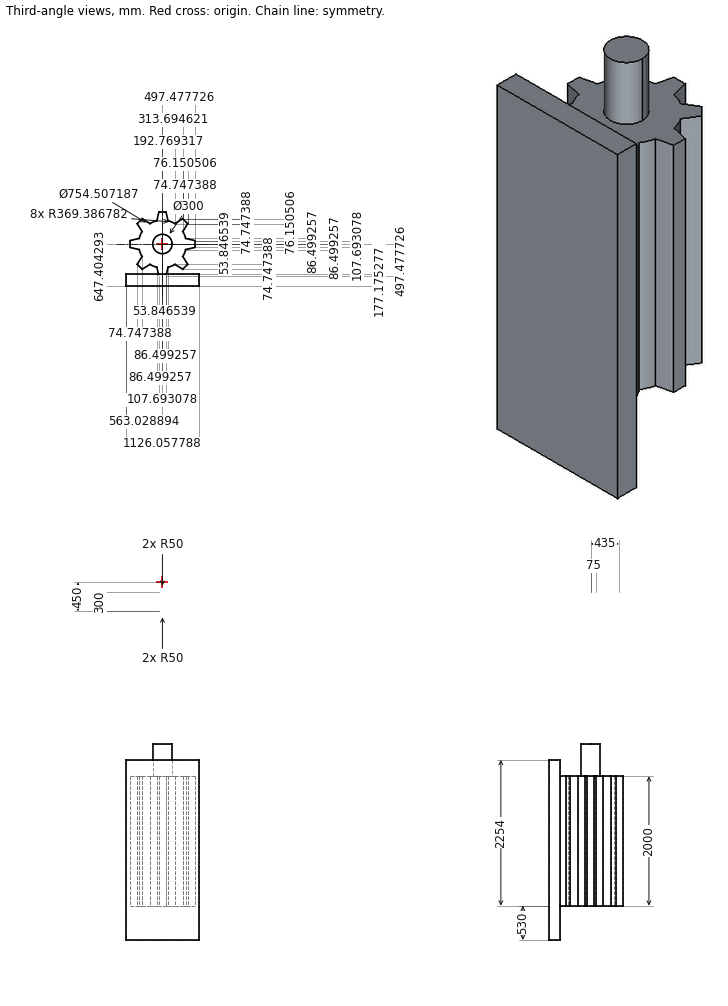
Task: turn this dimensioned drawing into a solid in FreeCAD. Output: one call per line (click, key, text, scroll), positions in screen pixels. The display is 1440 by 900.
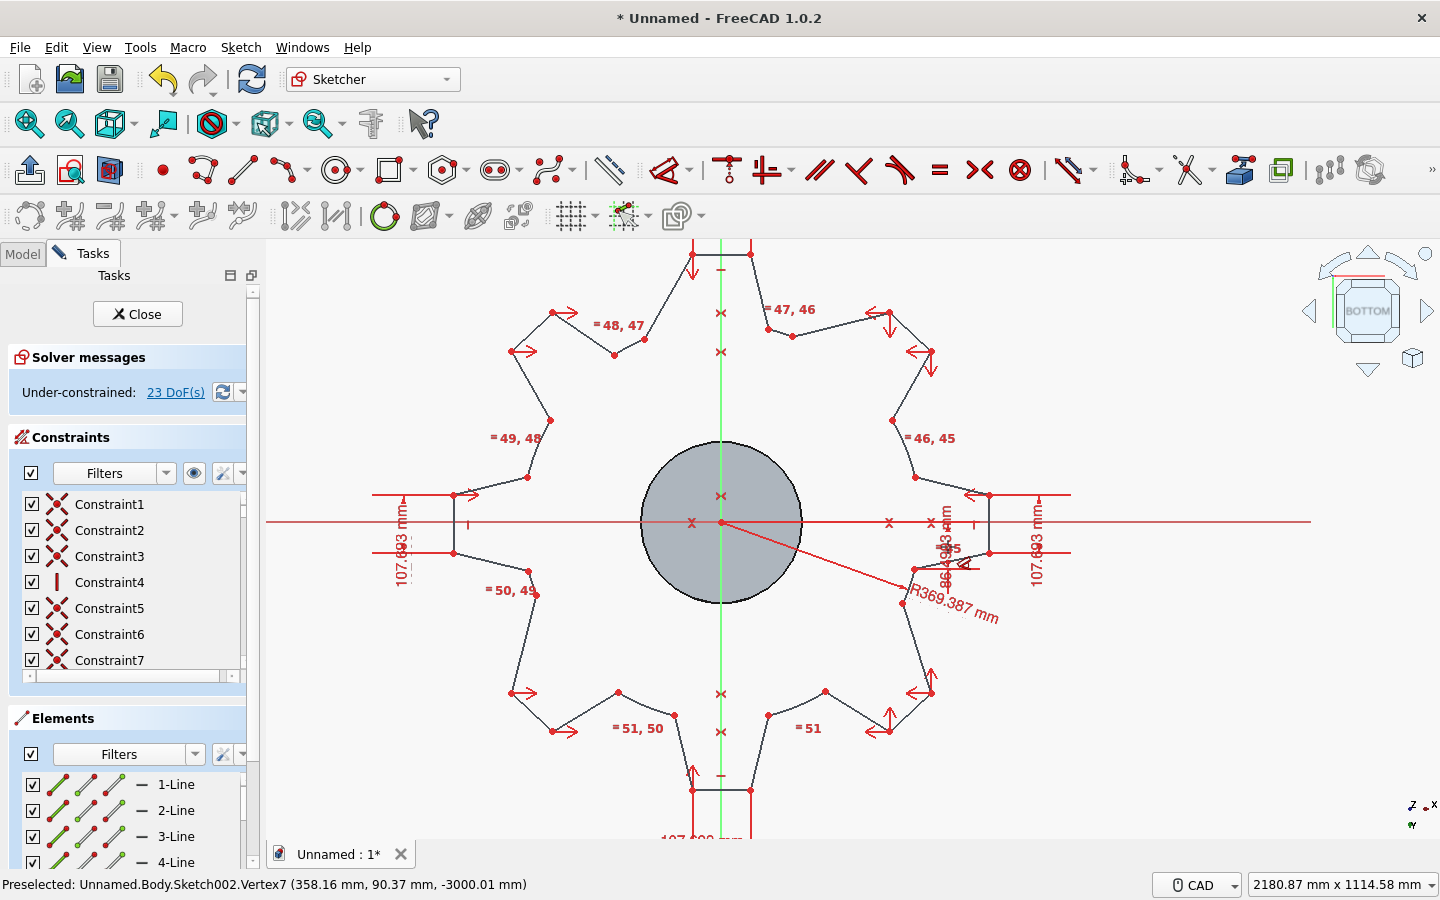
scroll(989, 553, up, 2)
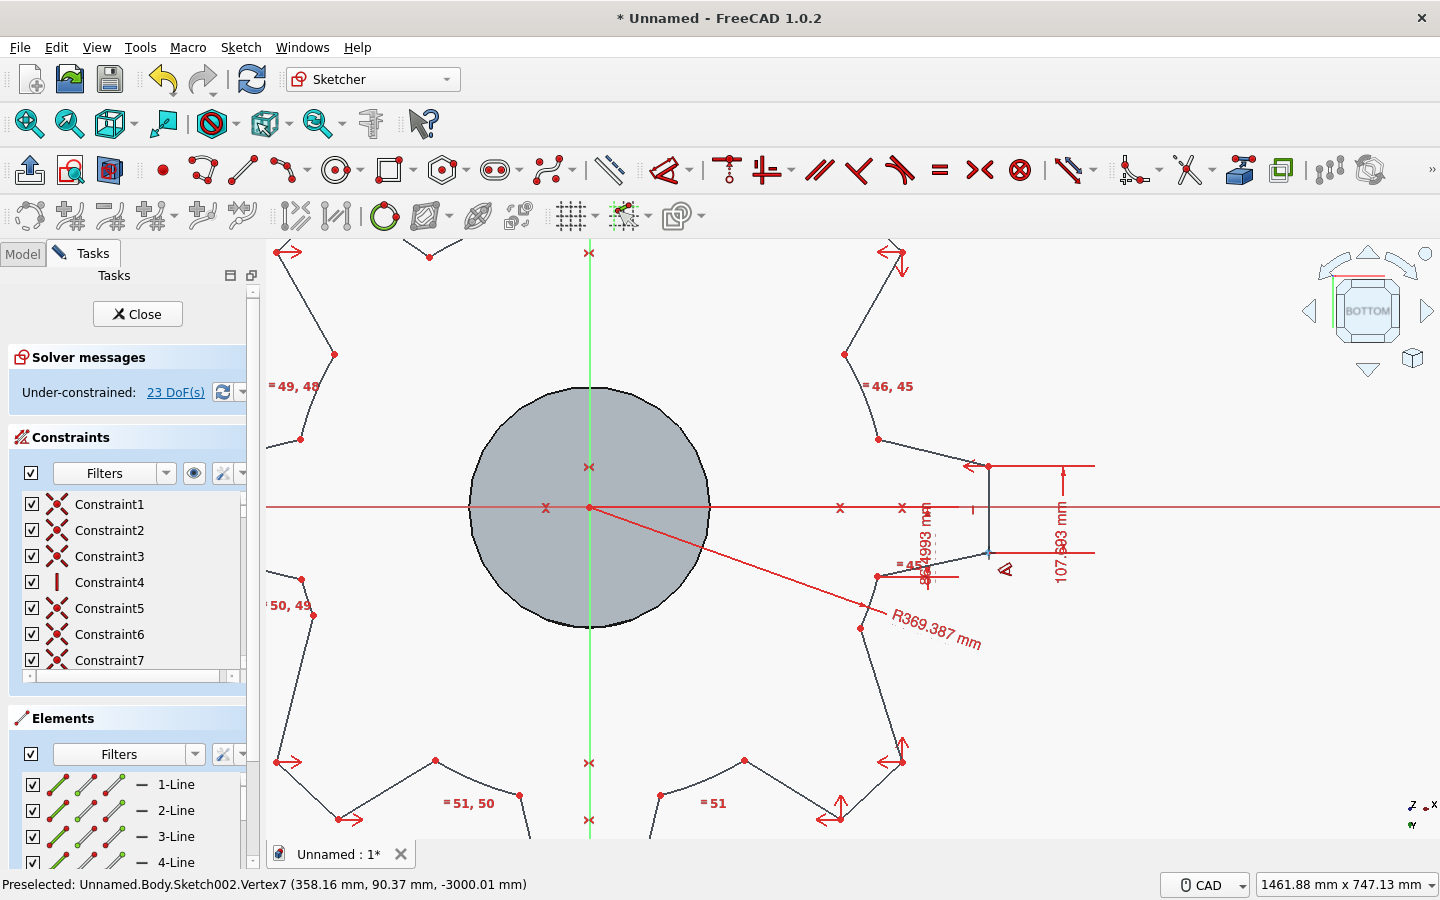
click(989, 553)
click(556, 530)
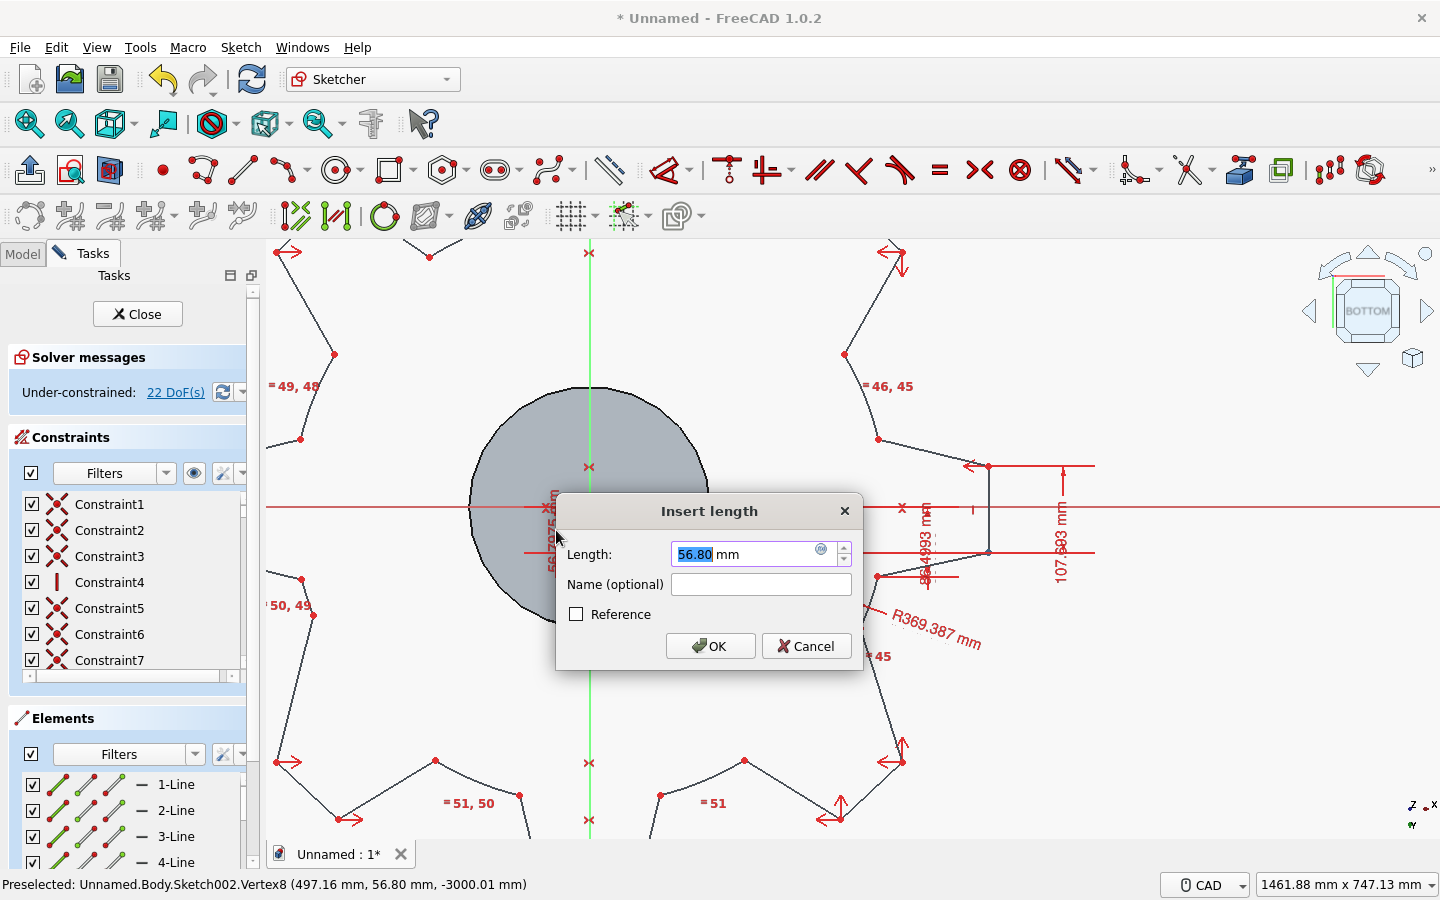
text(53.846539)
key(Return)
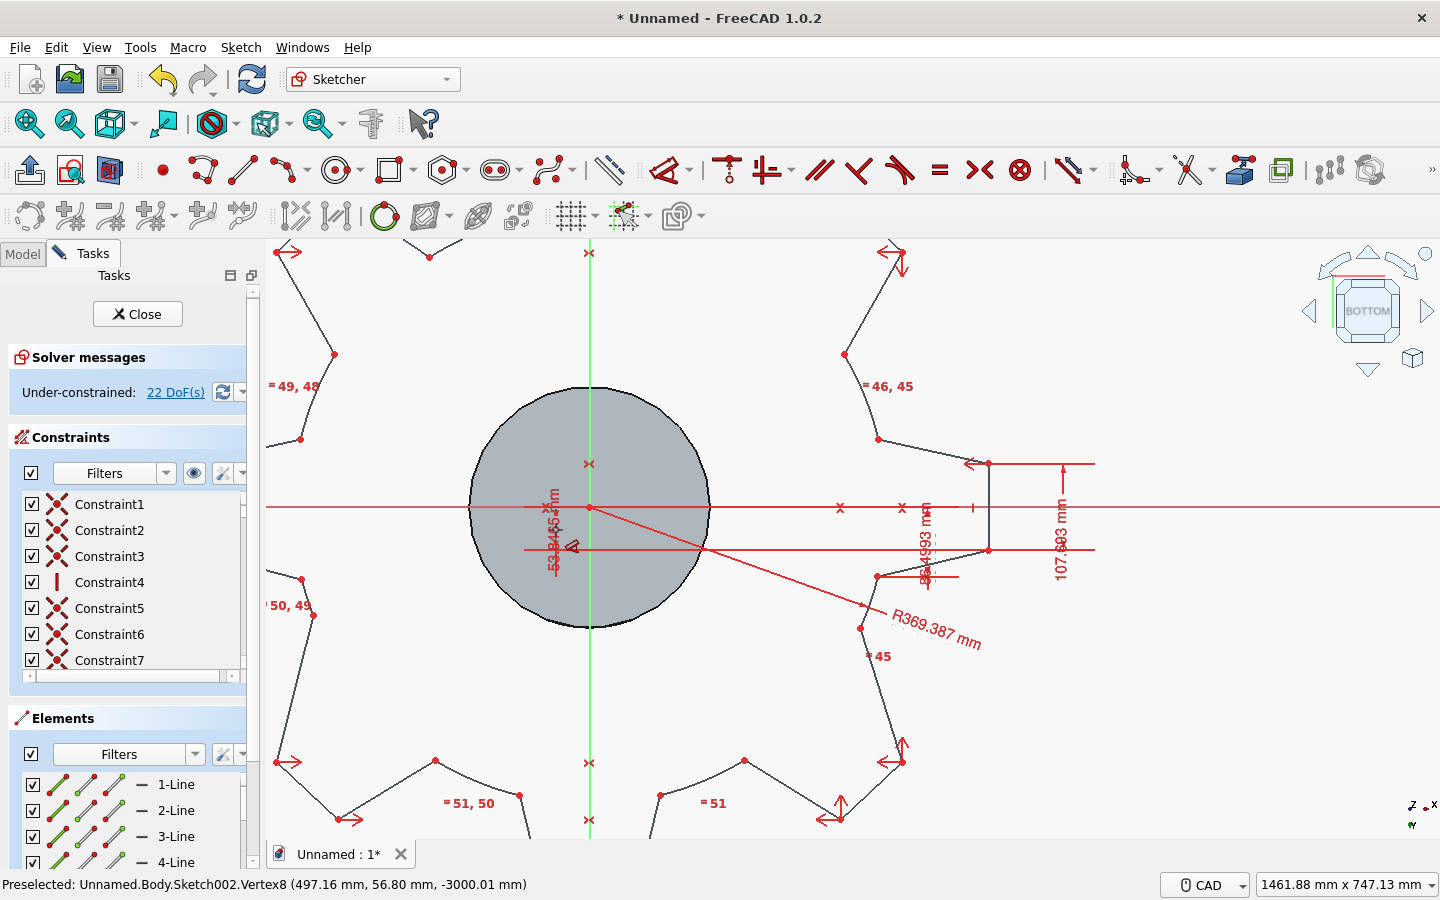
click(878, 440)
click(912, 473)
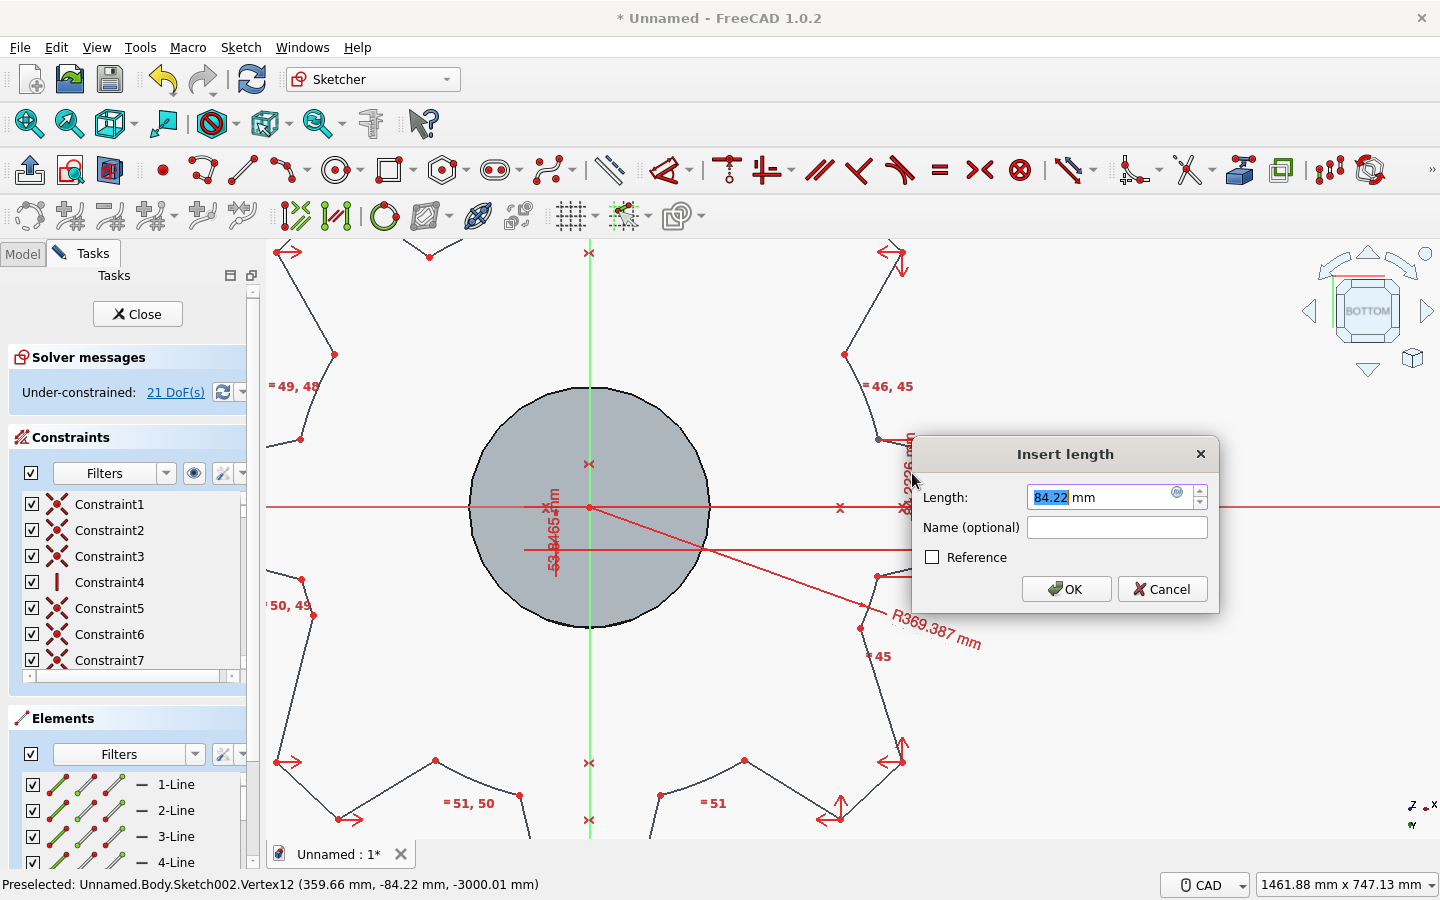
text(86.499257)
key(Return)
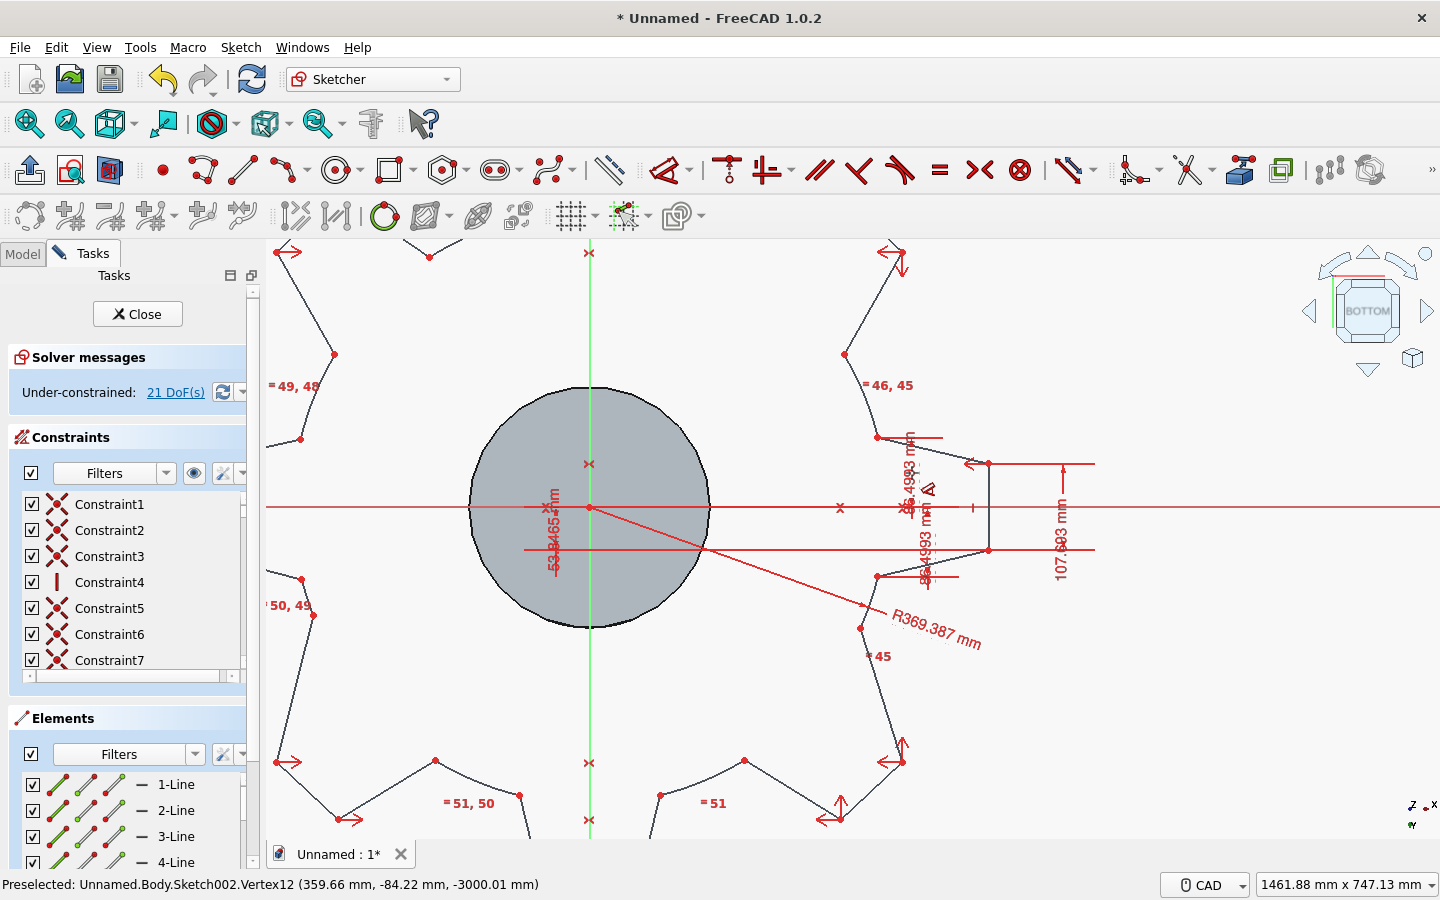
scroll(944, 565, down, 4)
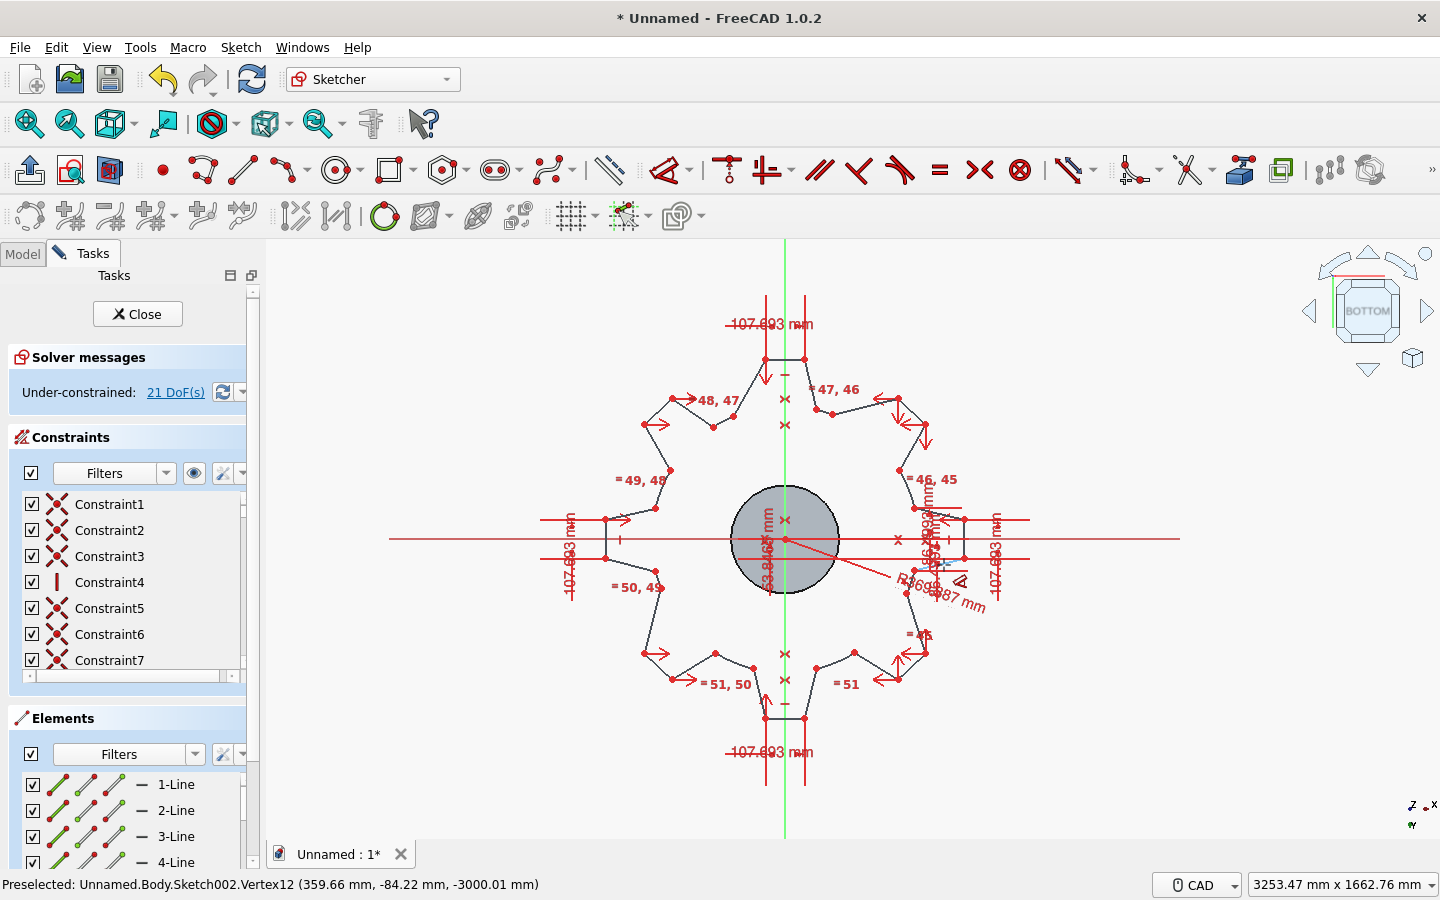
scroll(817, 410, up, 2)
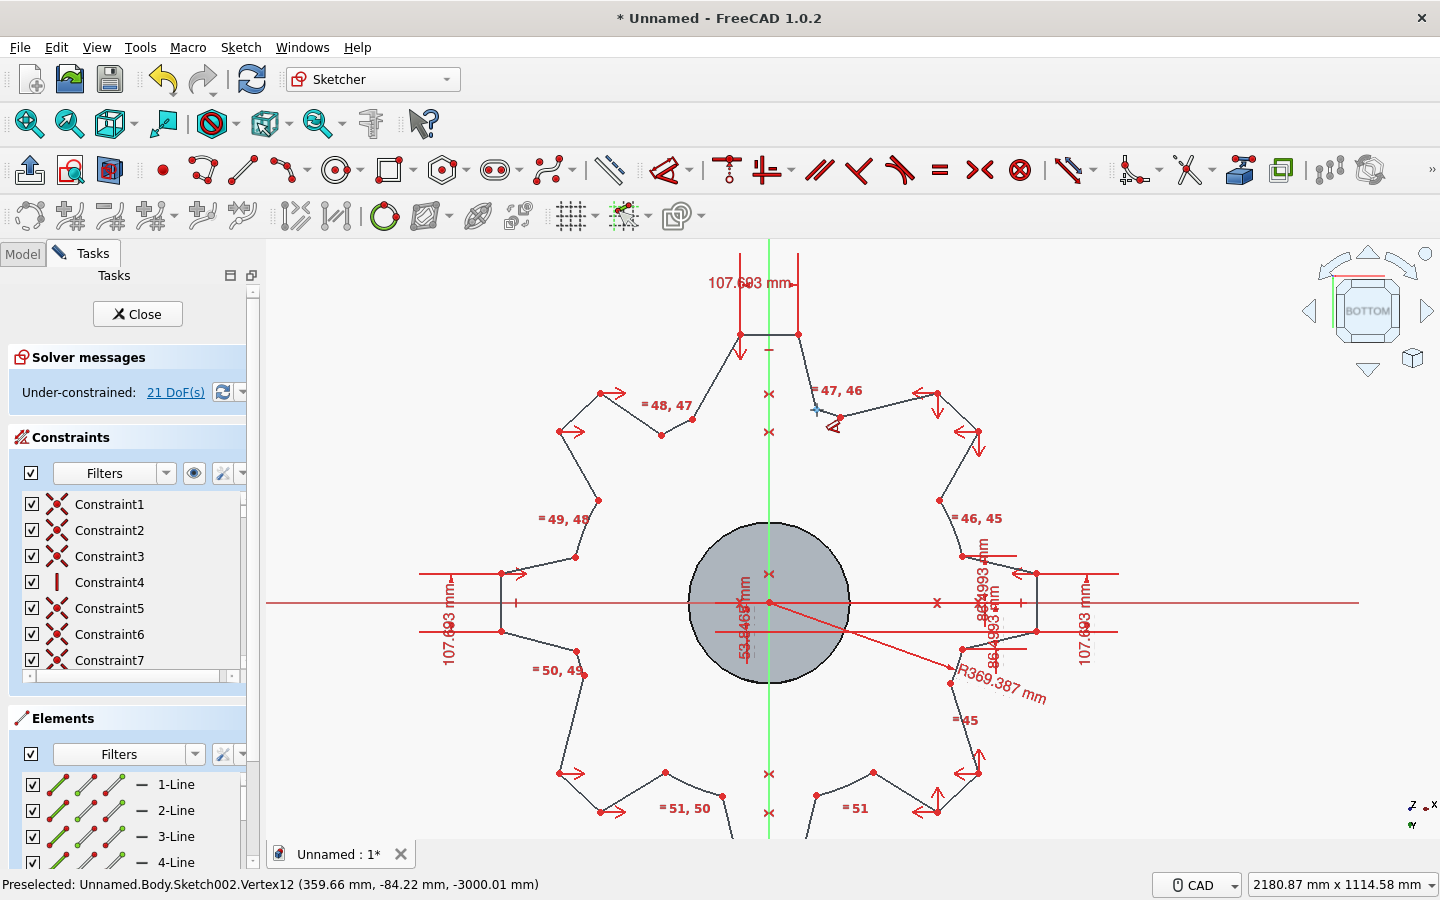
click(816, 410)
click(793, 376)